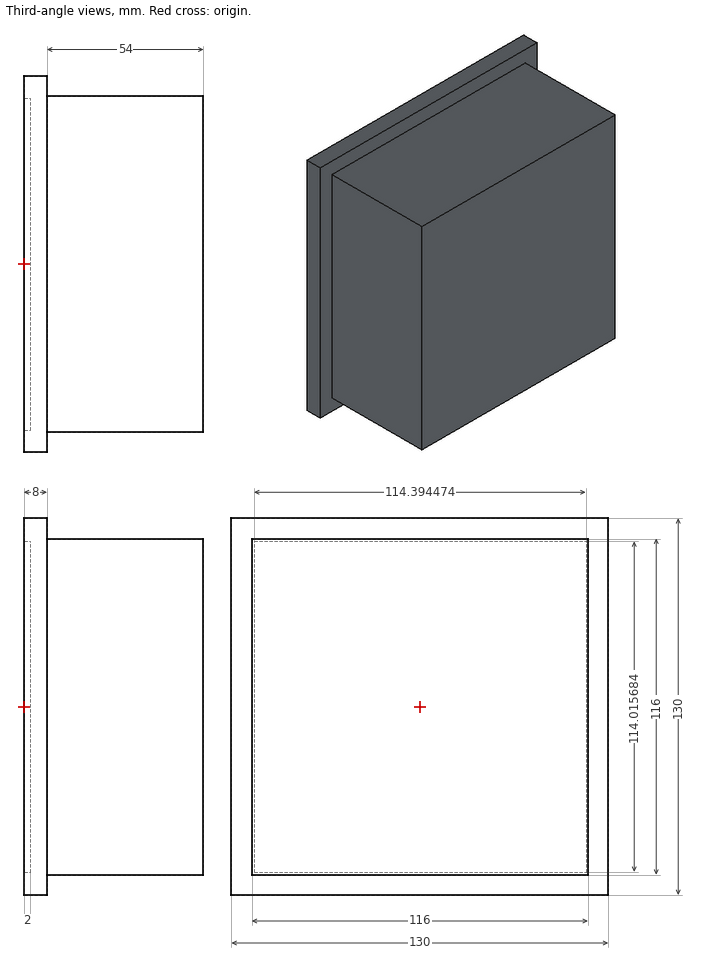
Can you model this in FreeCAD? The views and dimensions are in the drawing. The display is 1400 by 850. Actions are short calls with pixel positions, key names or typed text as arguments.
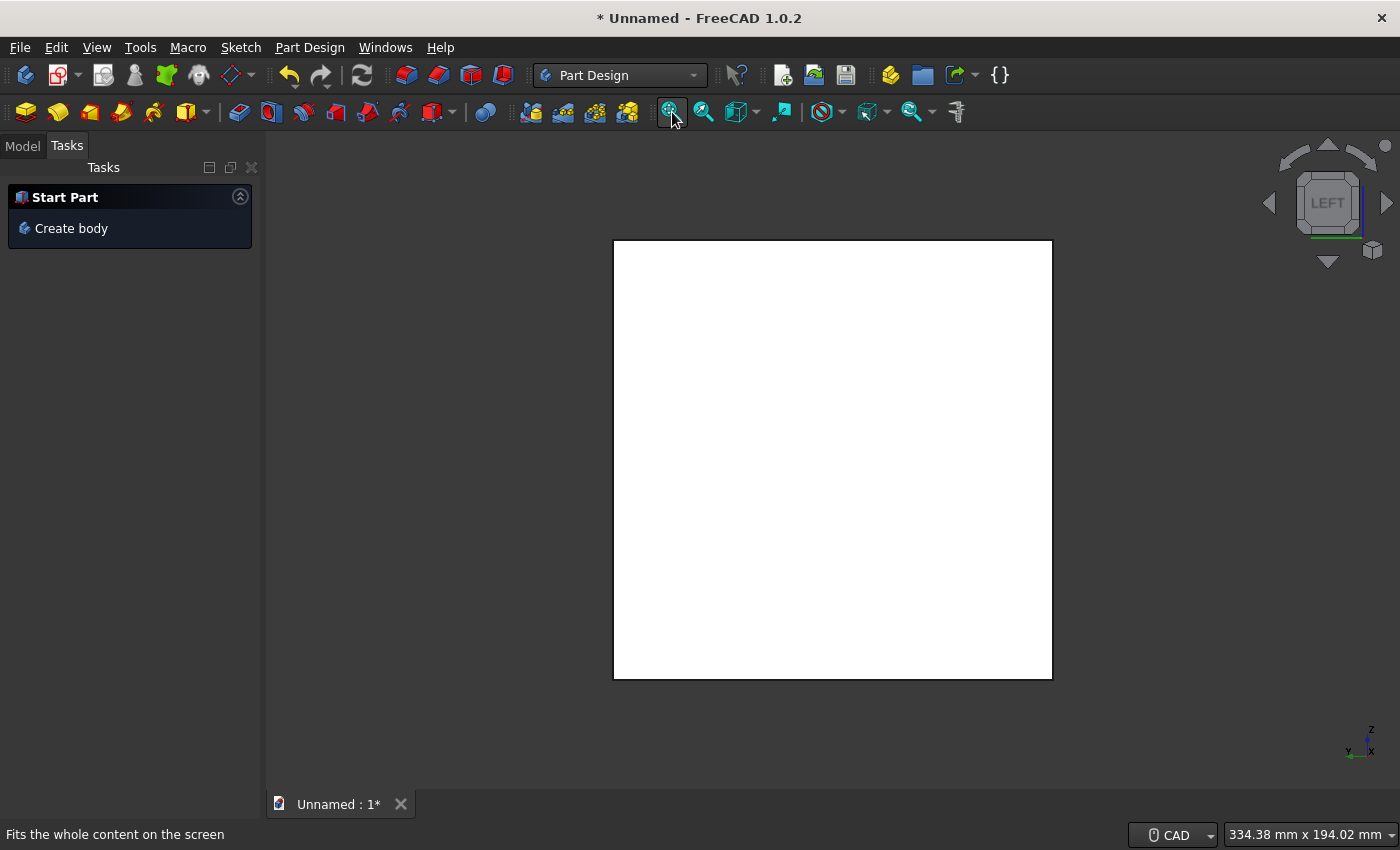
click(833, 459)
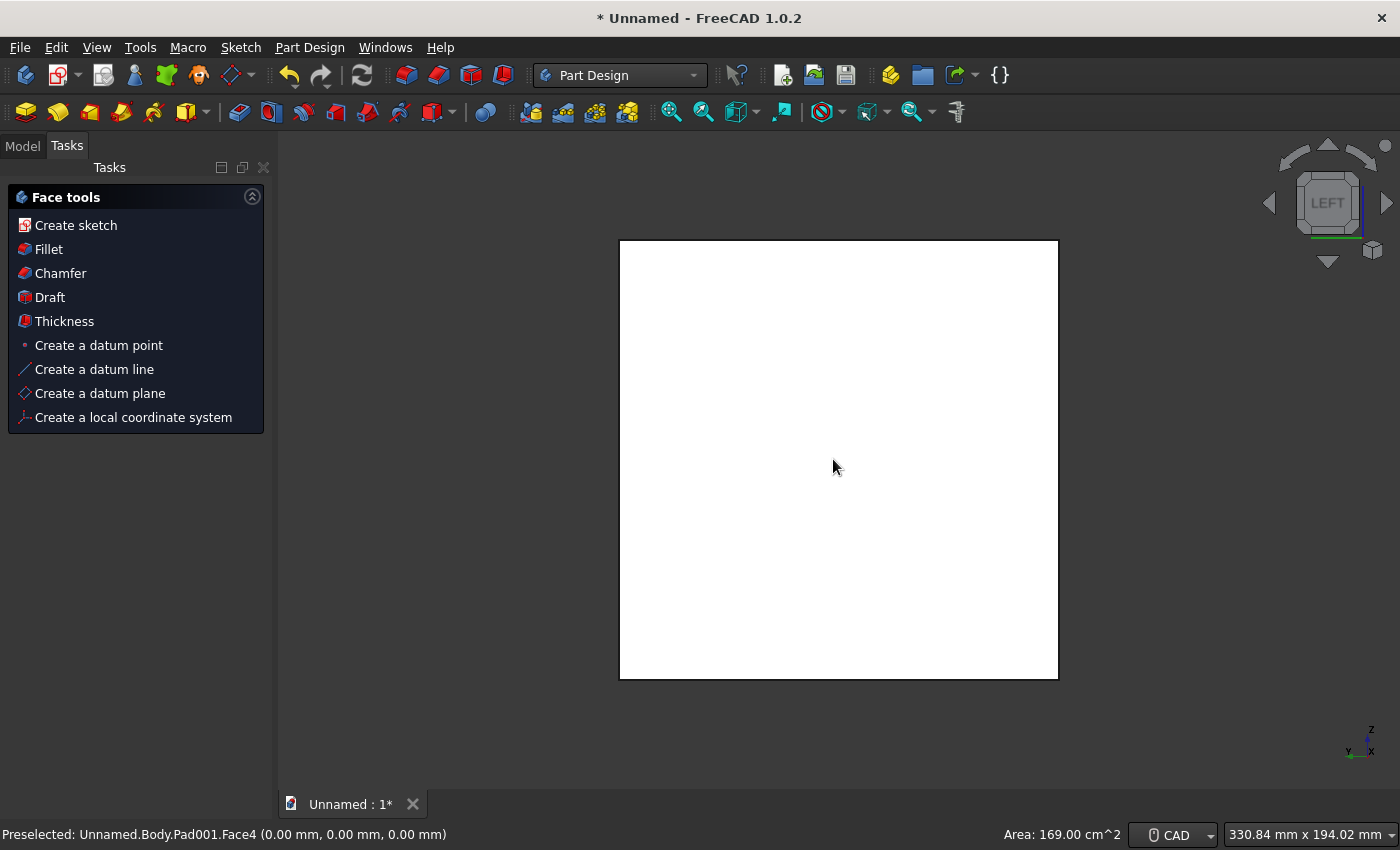
click(58, 76)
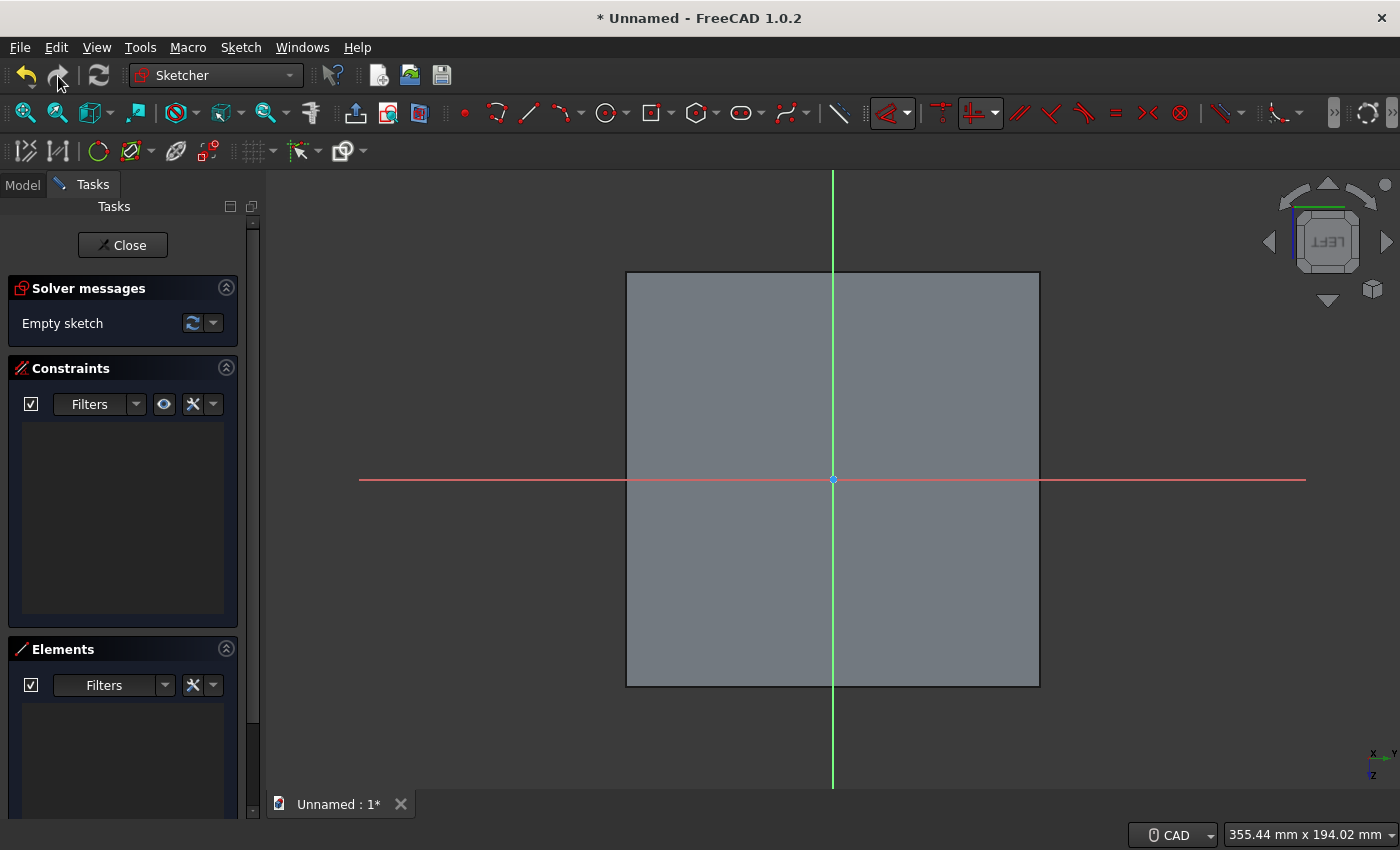
click(652, 114)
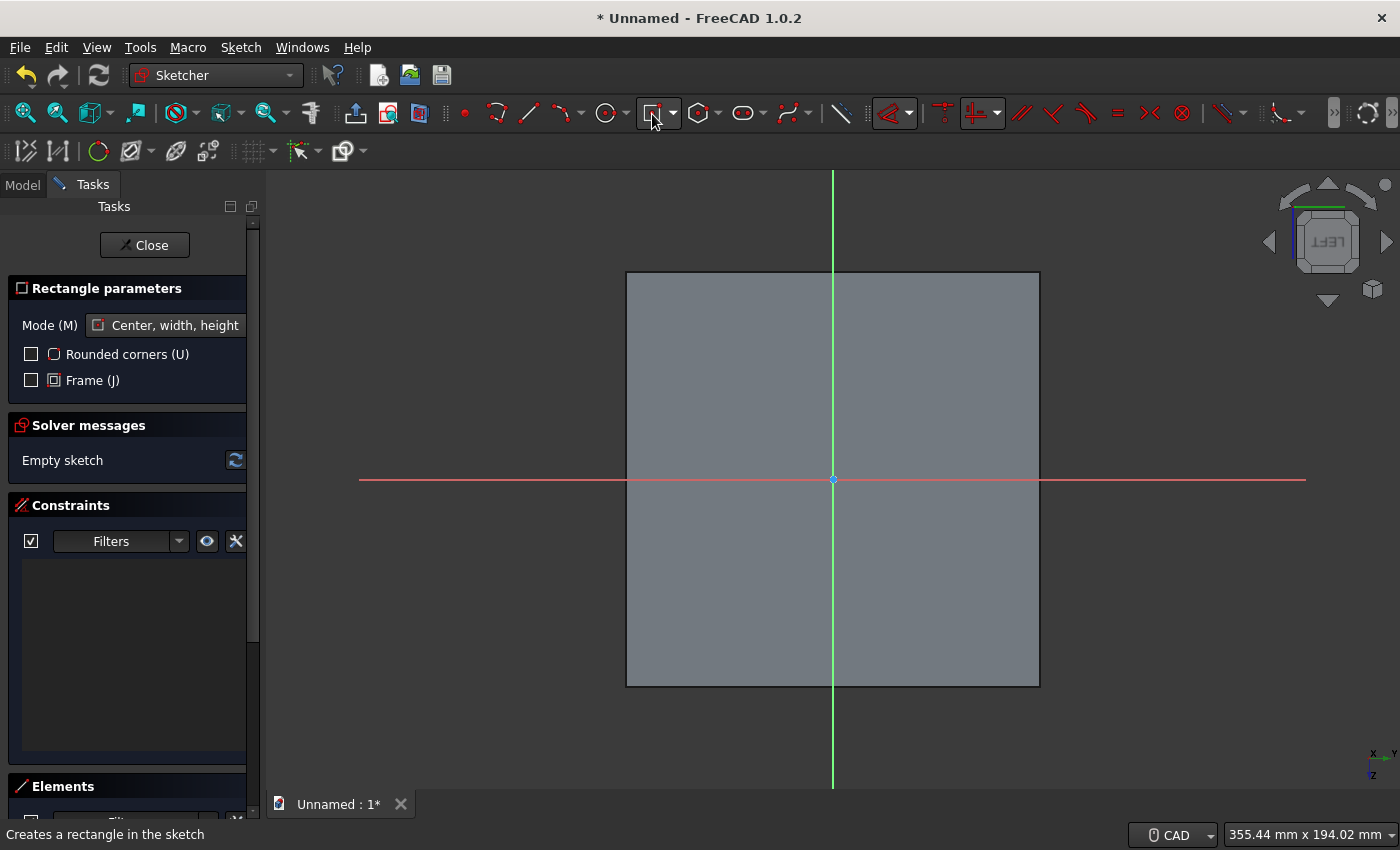
click(833, 480)
click(1015, 298)
key(Escape)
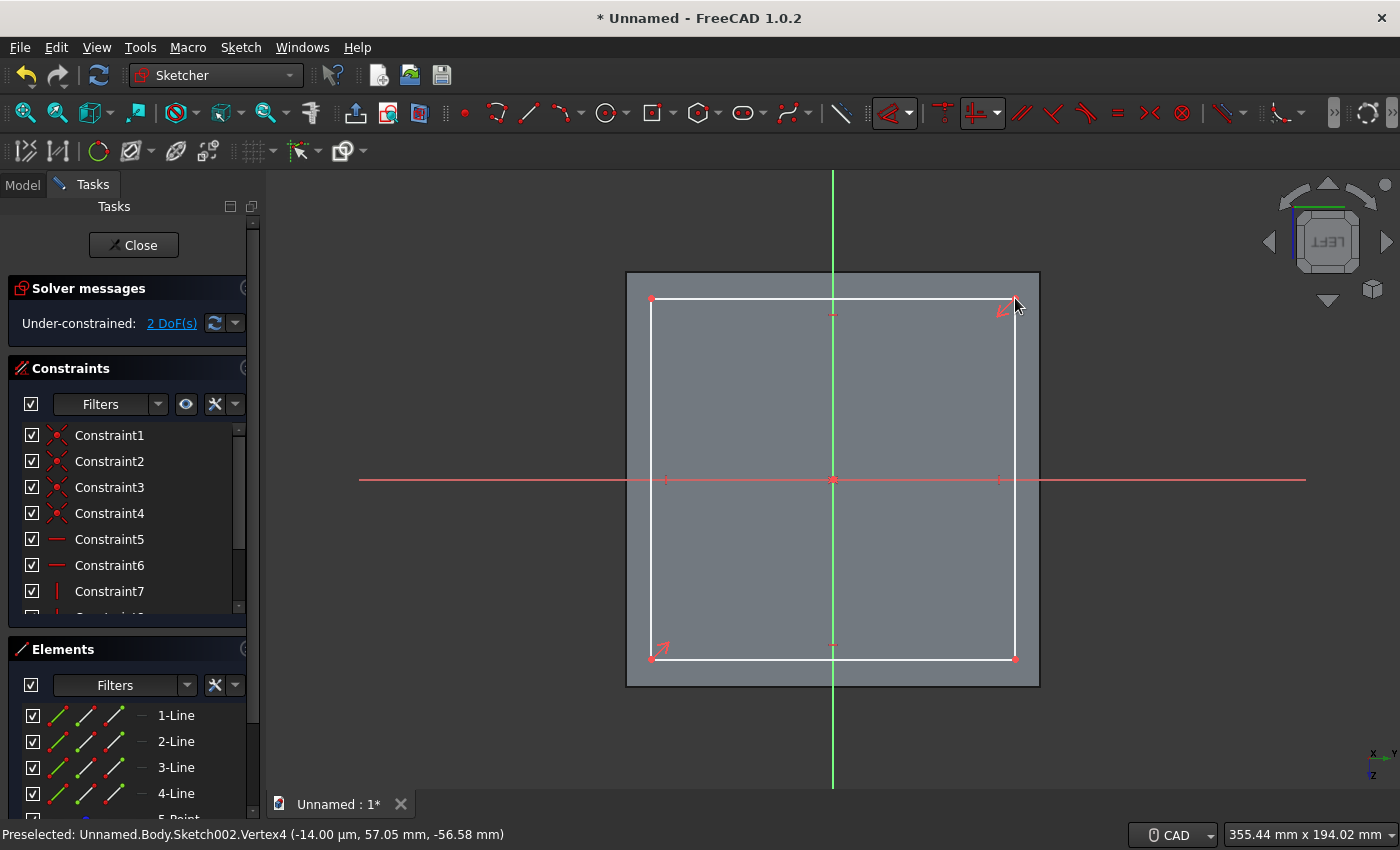
click(760, 660)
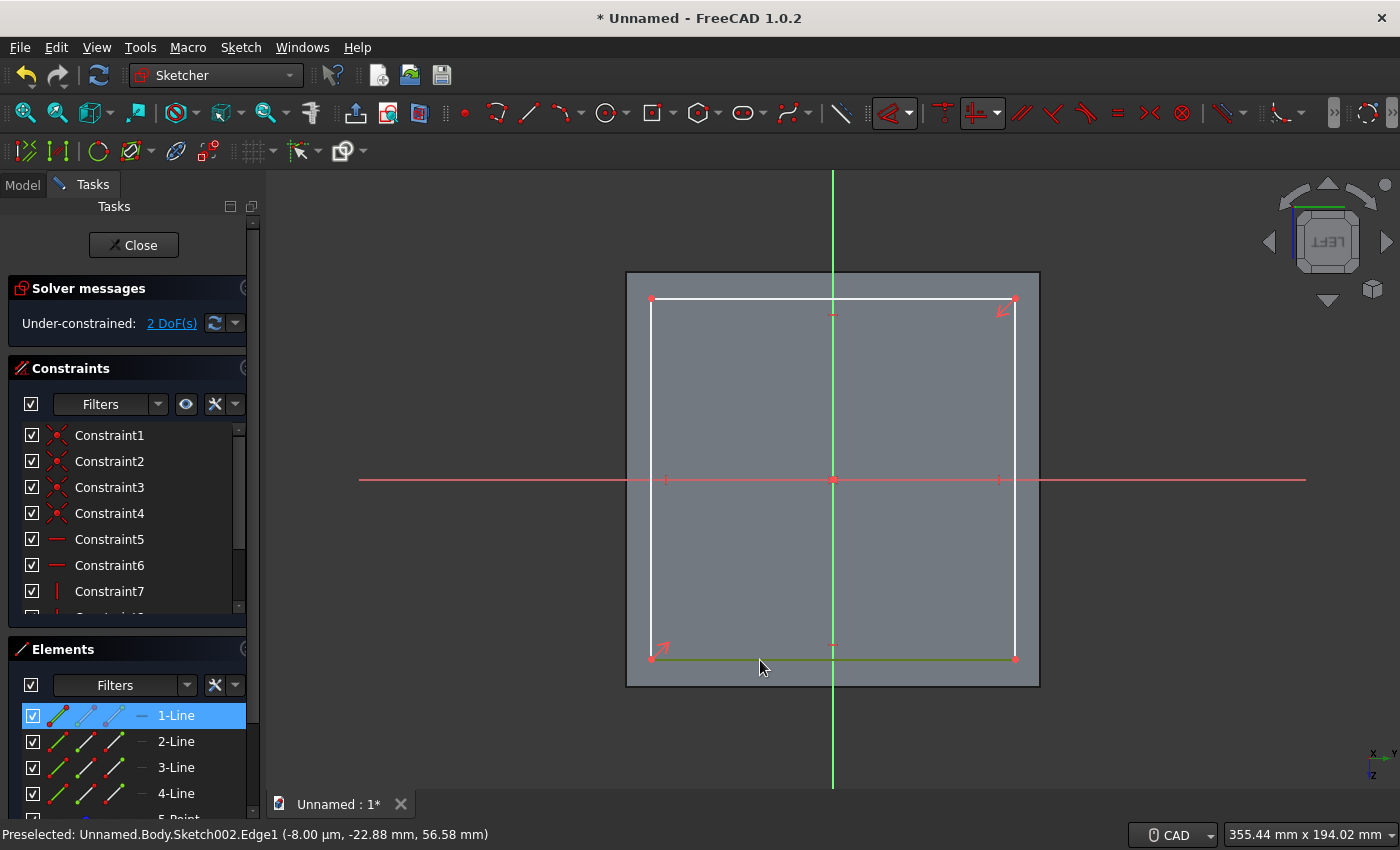
click(912, 114)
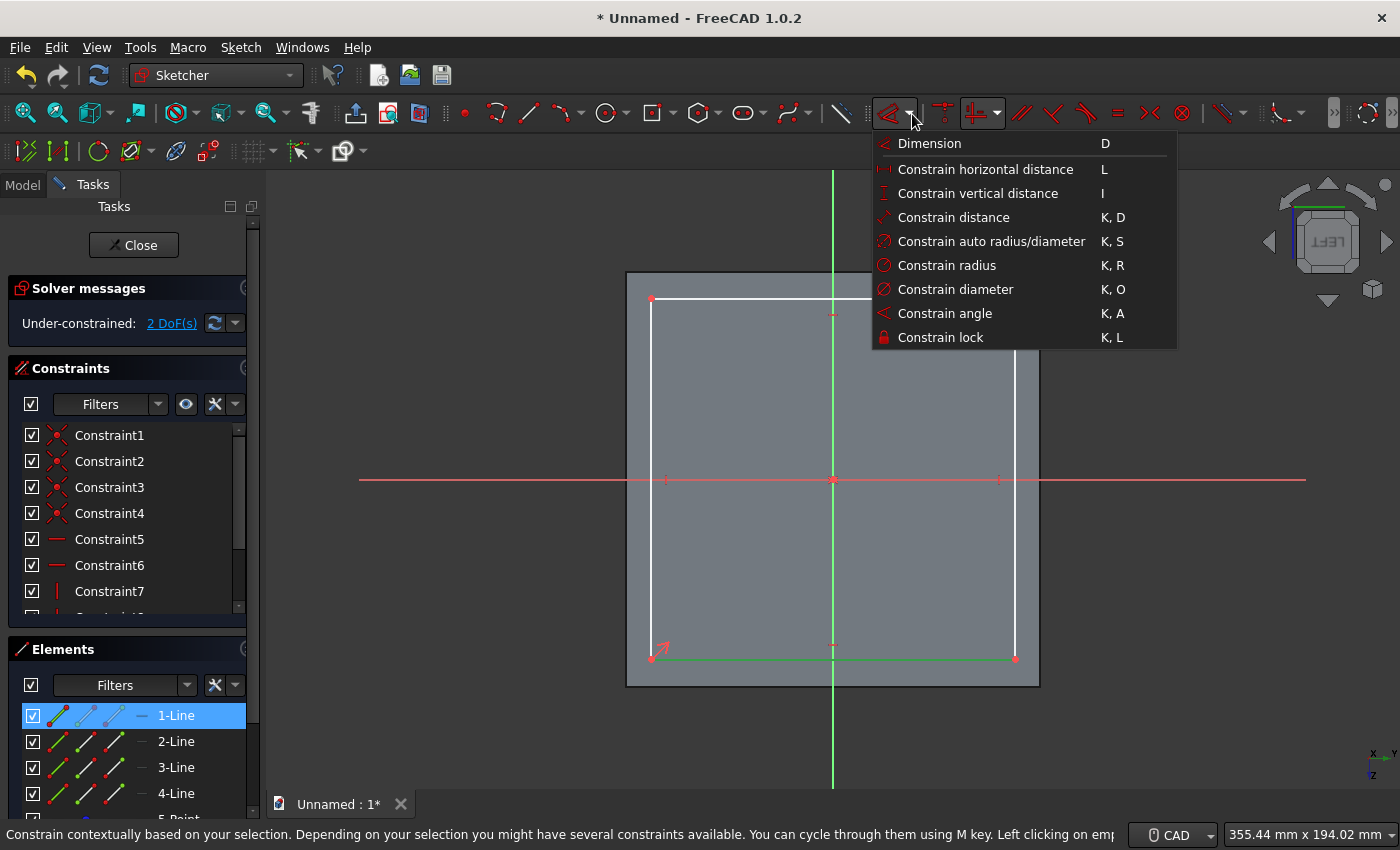
click(1025, 169)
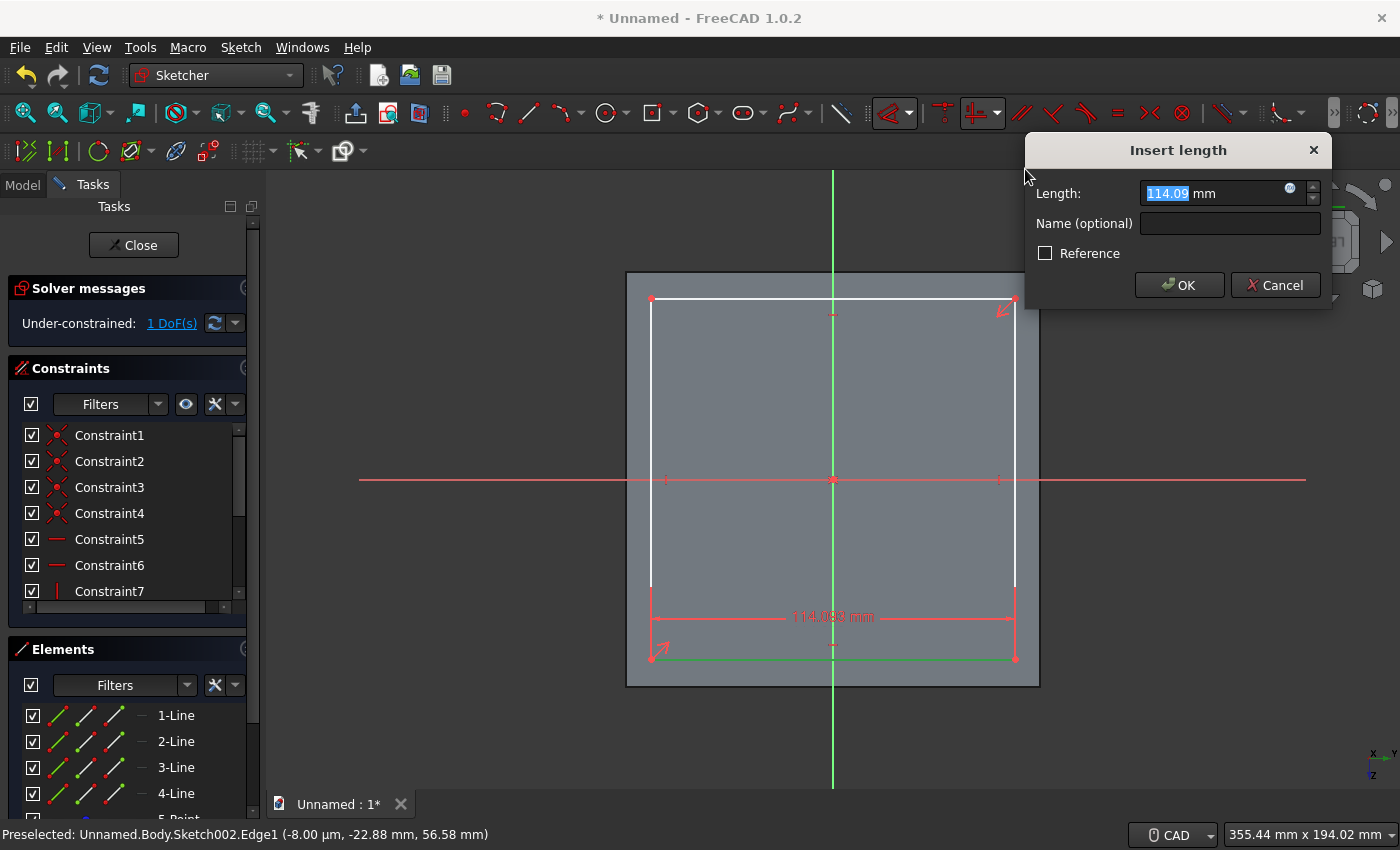
text(114.394474)
key(Return)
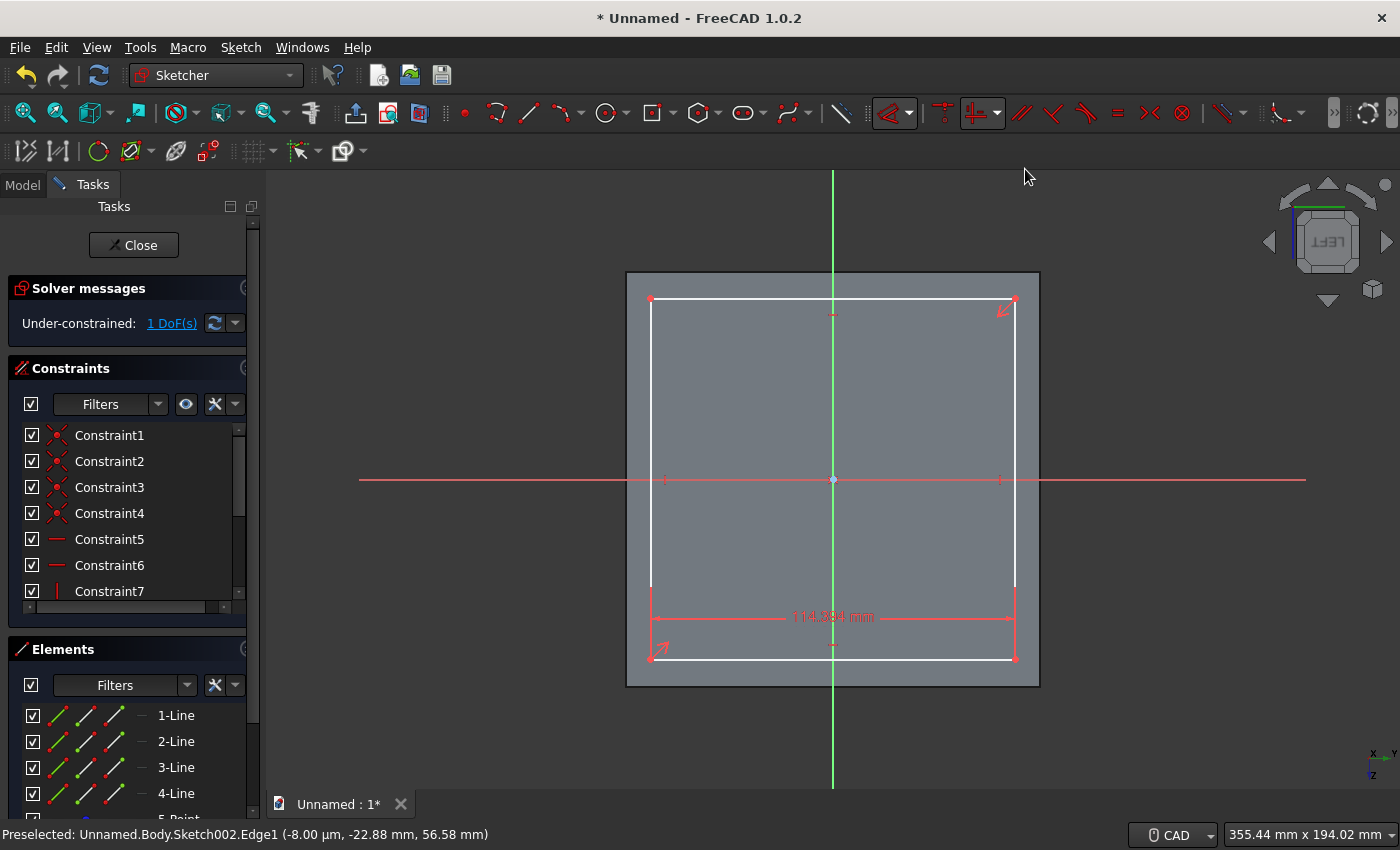
click(1015, 552)